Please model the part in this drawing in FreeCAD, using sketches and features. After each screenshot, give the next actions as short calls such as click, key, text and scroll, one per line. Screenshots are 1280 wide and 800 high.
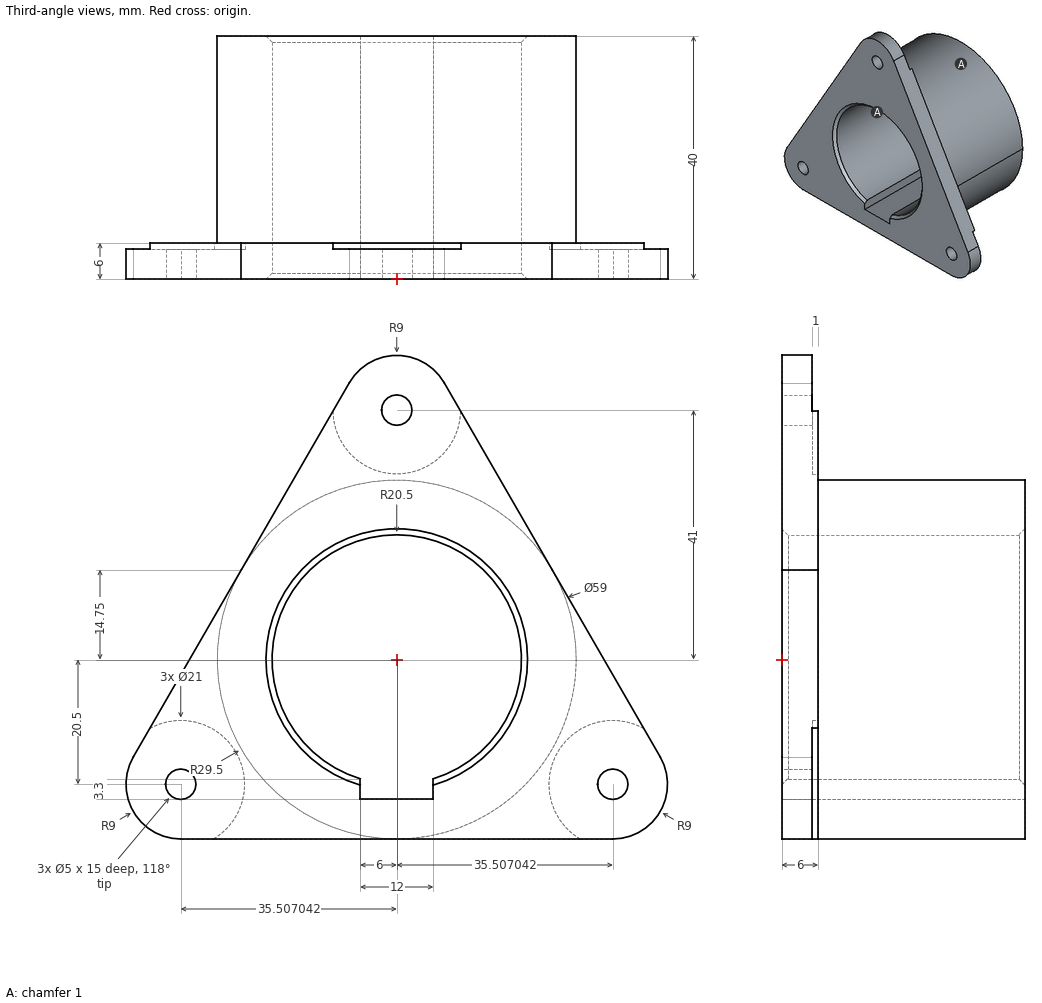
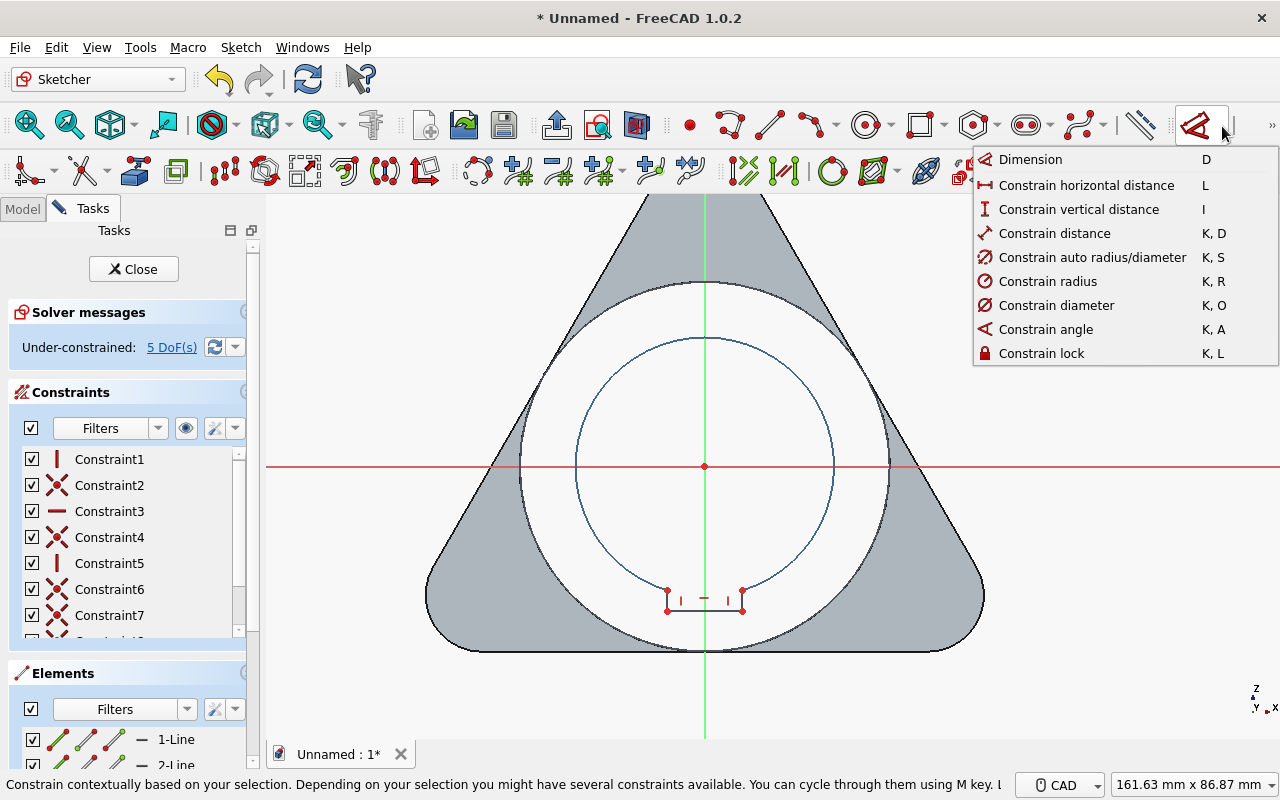
click(1126, 281)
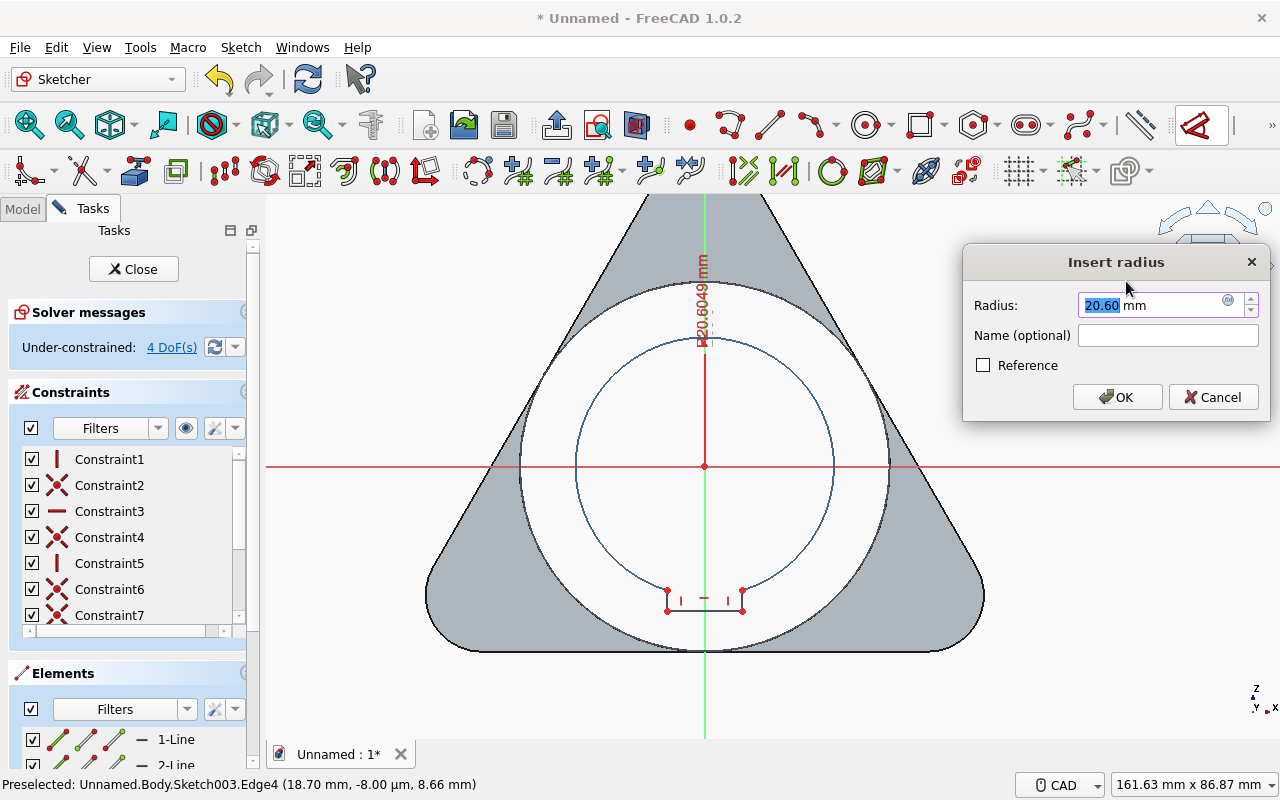
text(20.5)
key(Return)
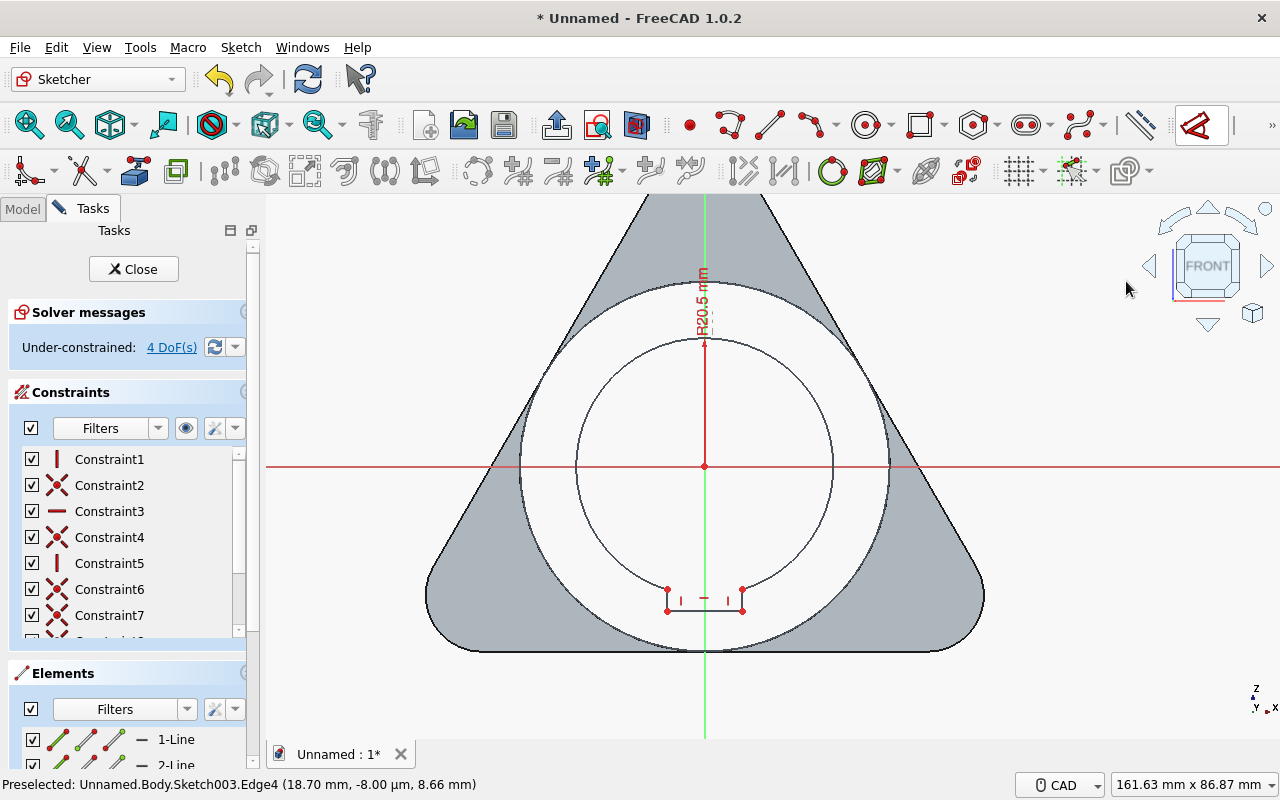
click(835, 336)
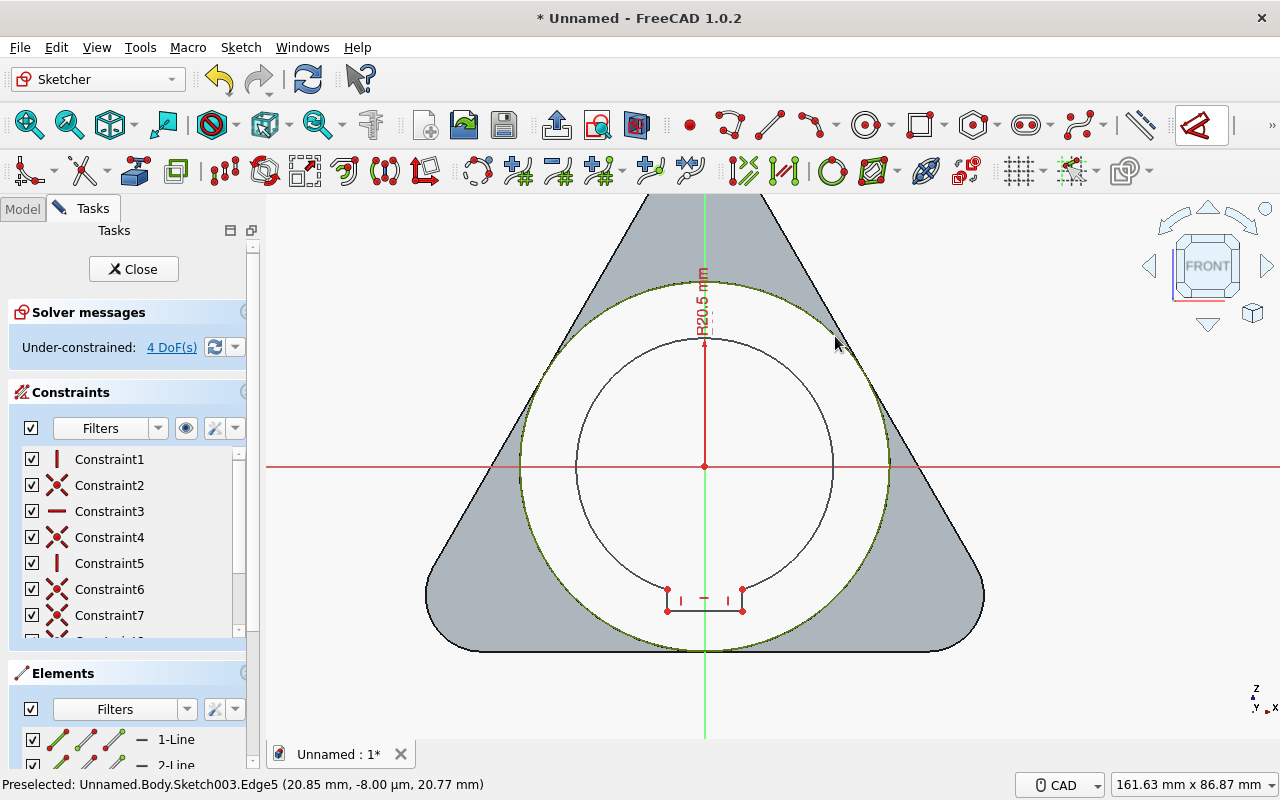
click(1222, 126)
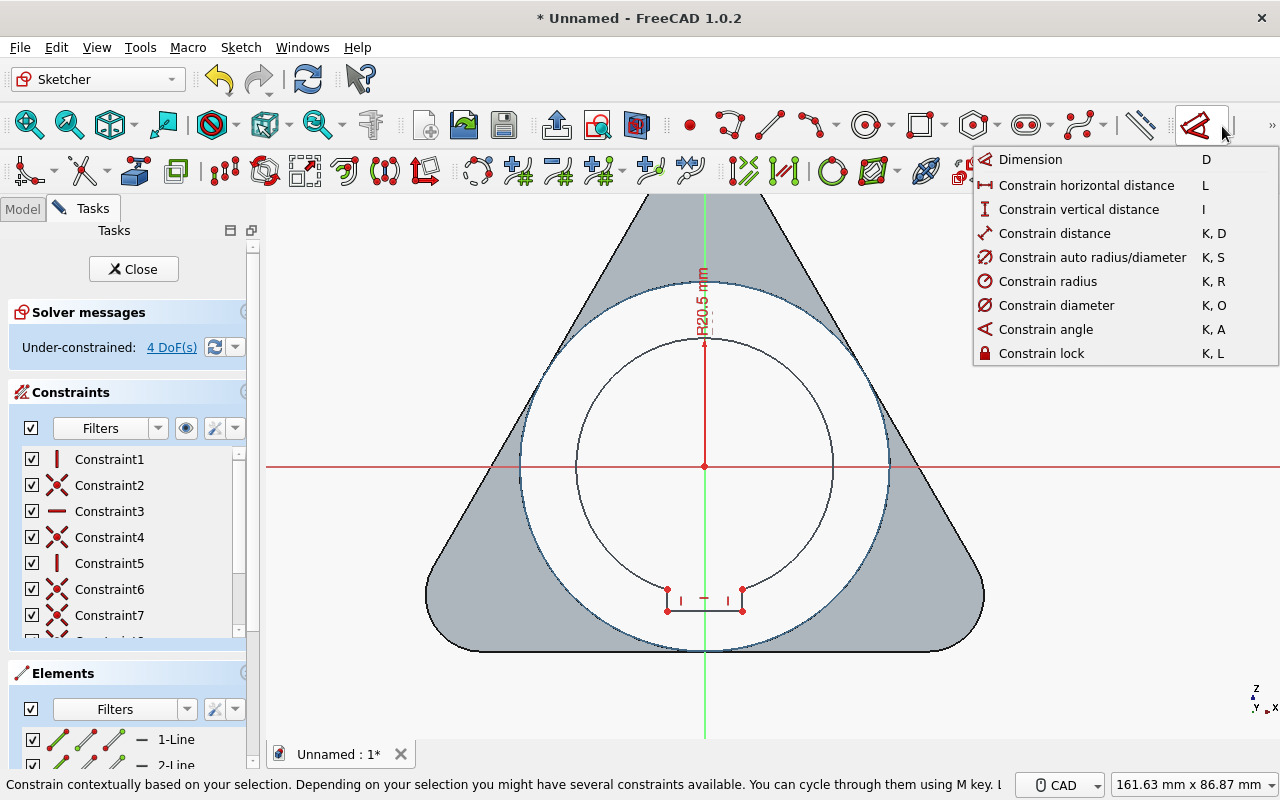
click(1126, 305)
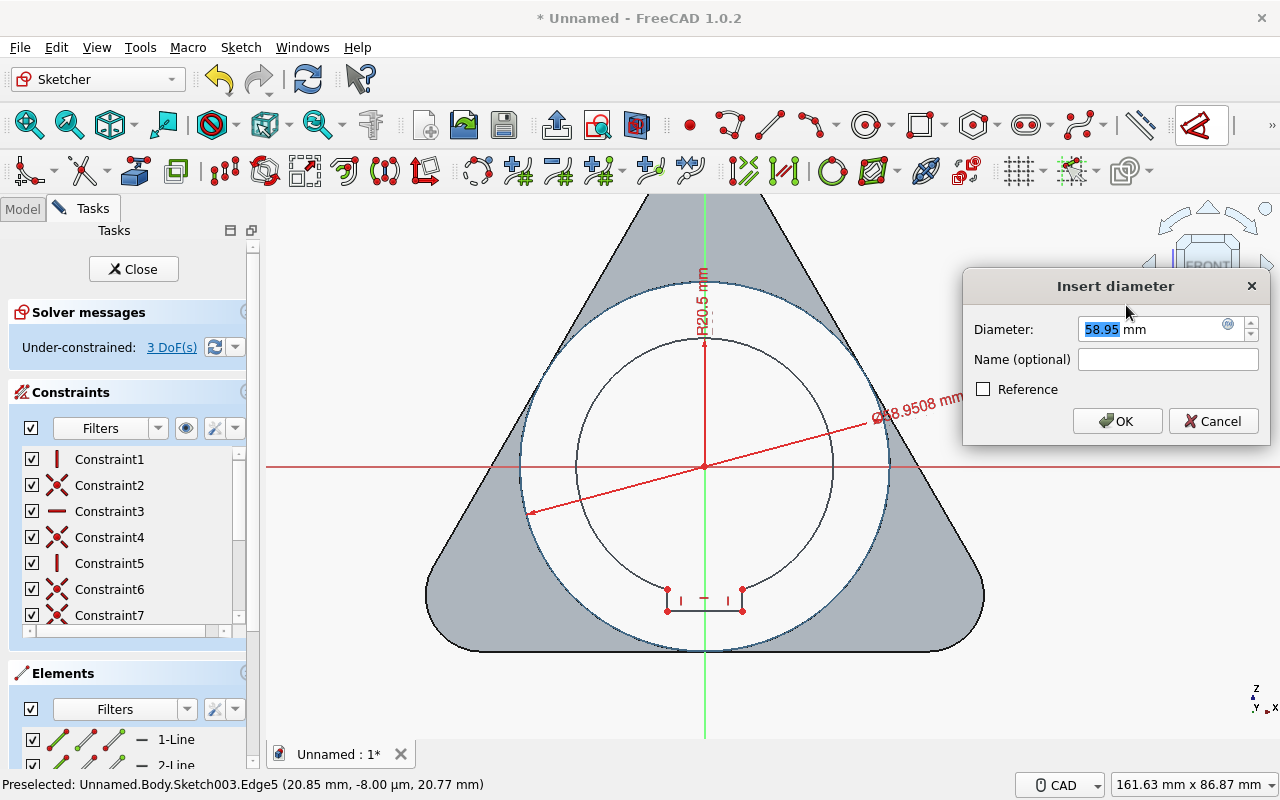
text(59)
key(Return)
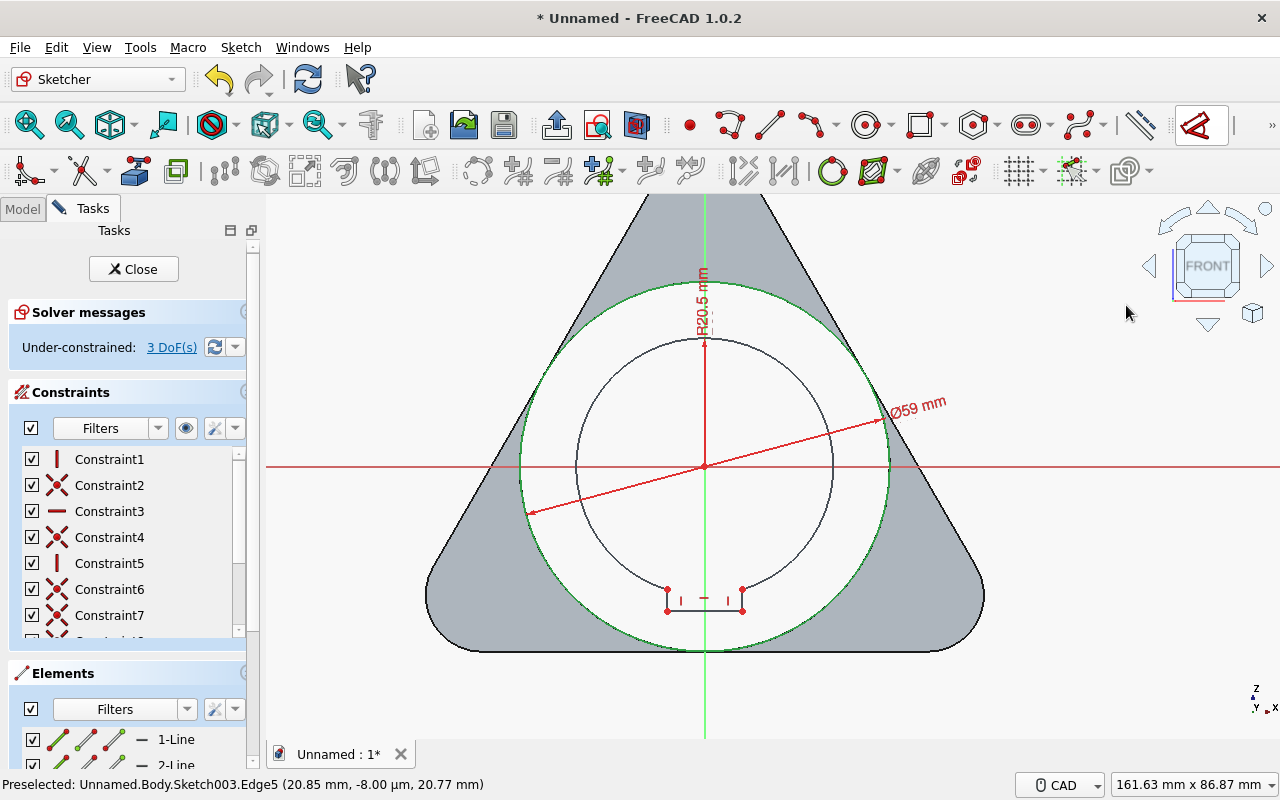
click(690, 611)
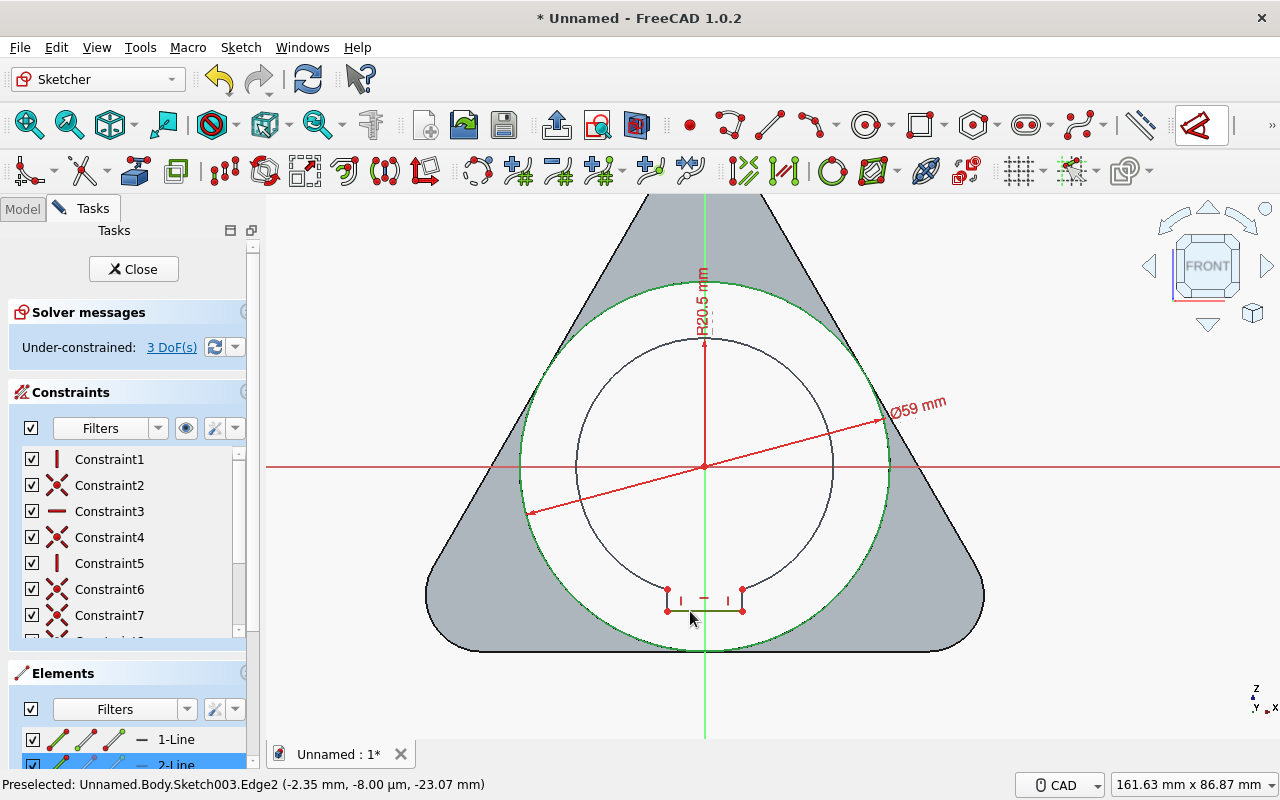
click(1222, 126)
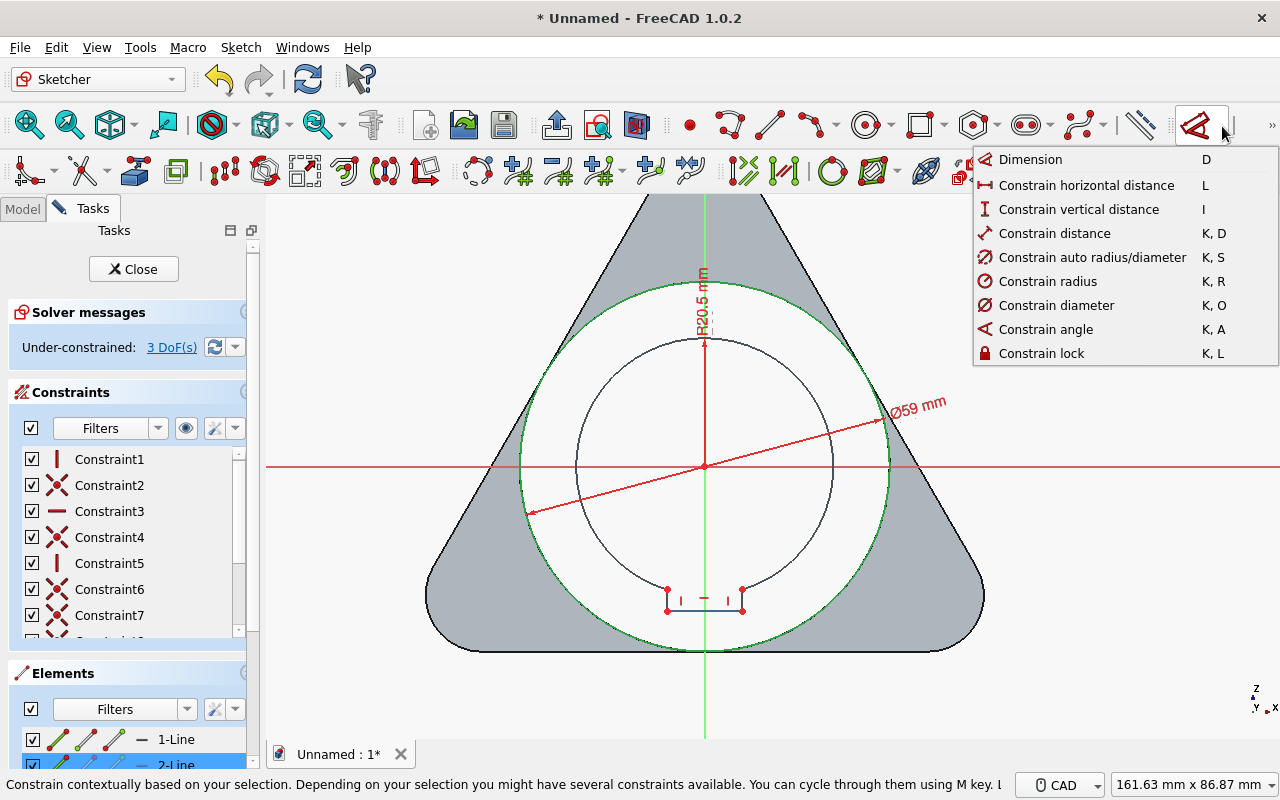
click(1126, 185)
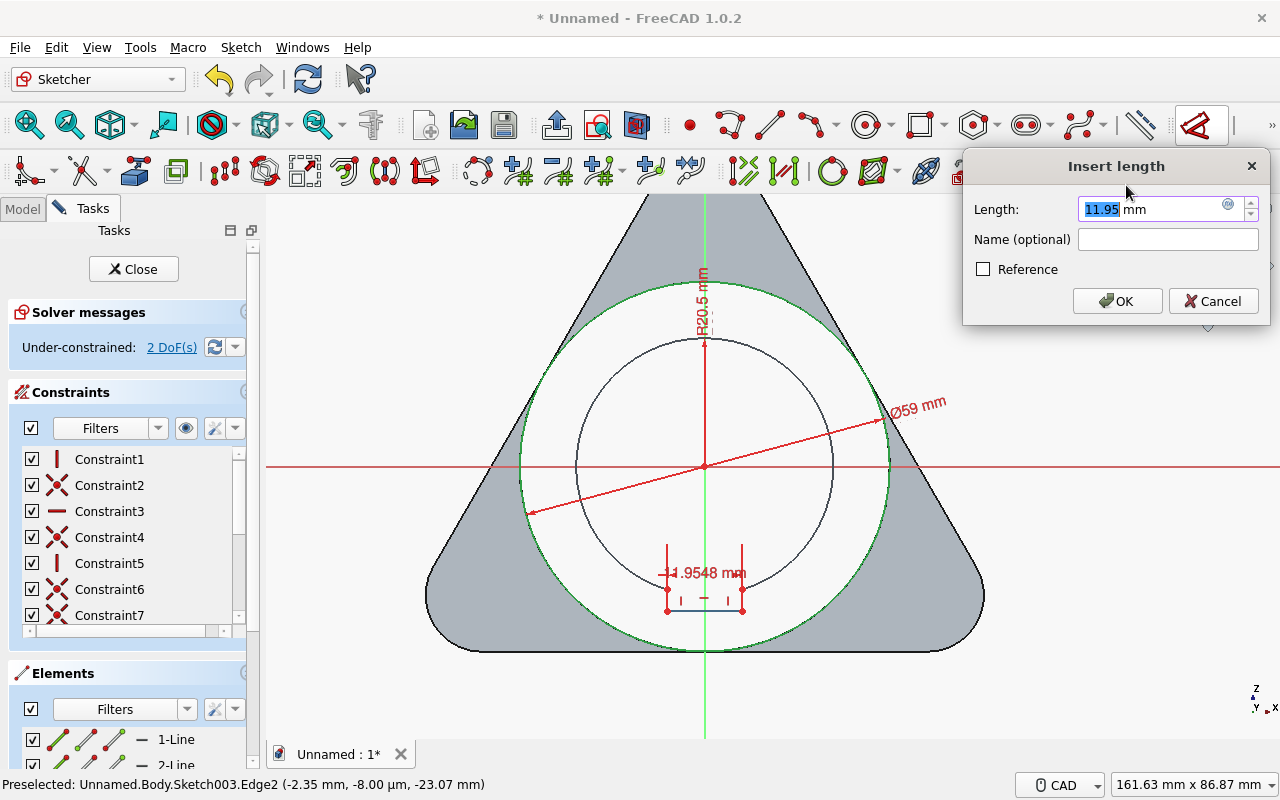
text(12)
key(Return)